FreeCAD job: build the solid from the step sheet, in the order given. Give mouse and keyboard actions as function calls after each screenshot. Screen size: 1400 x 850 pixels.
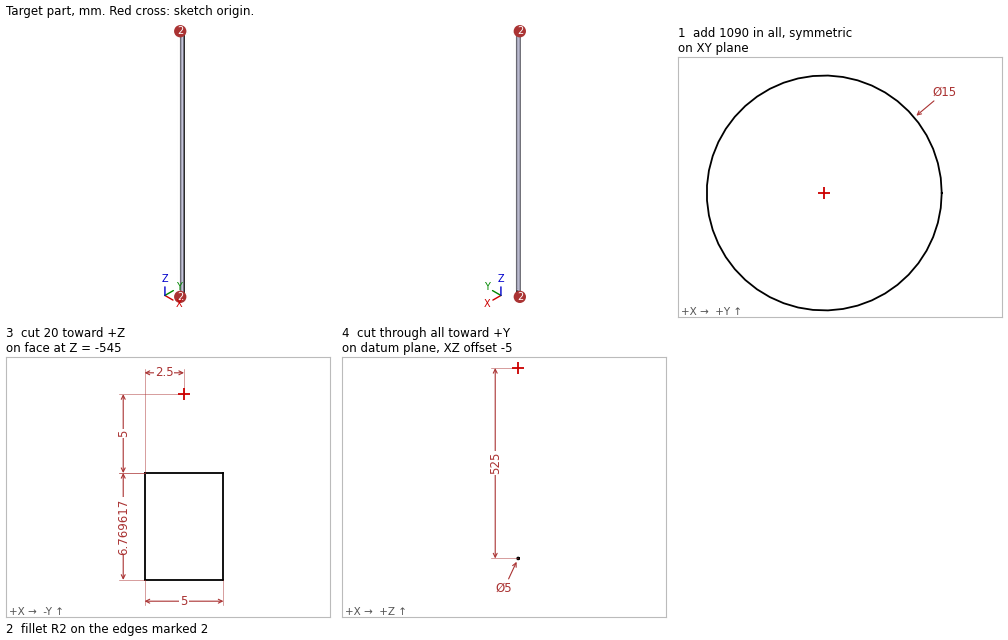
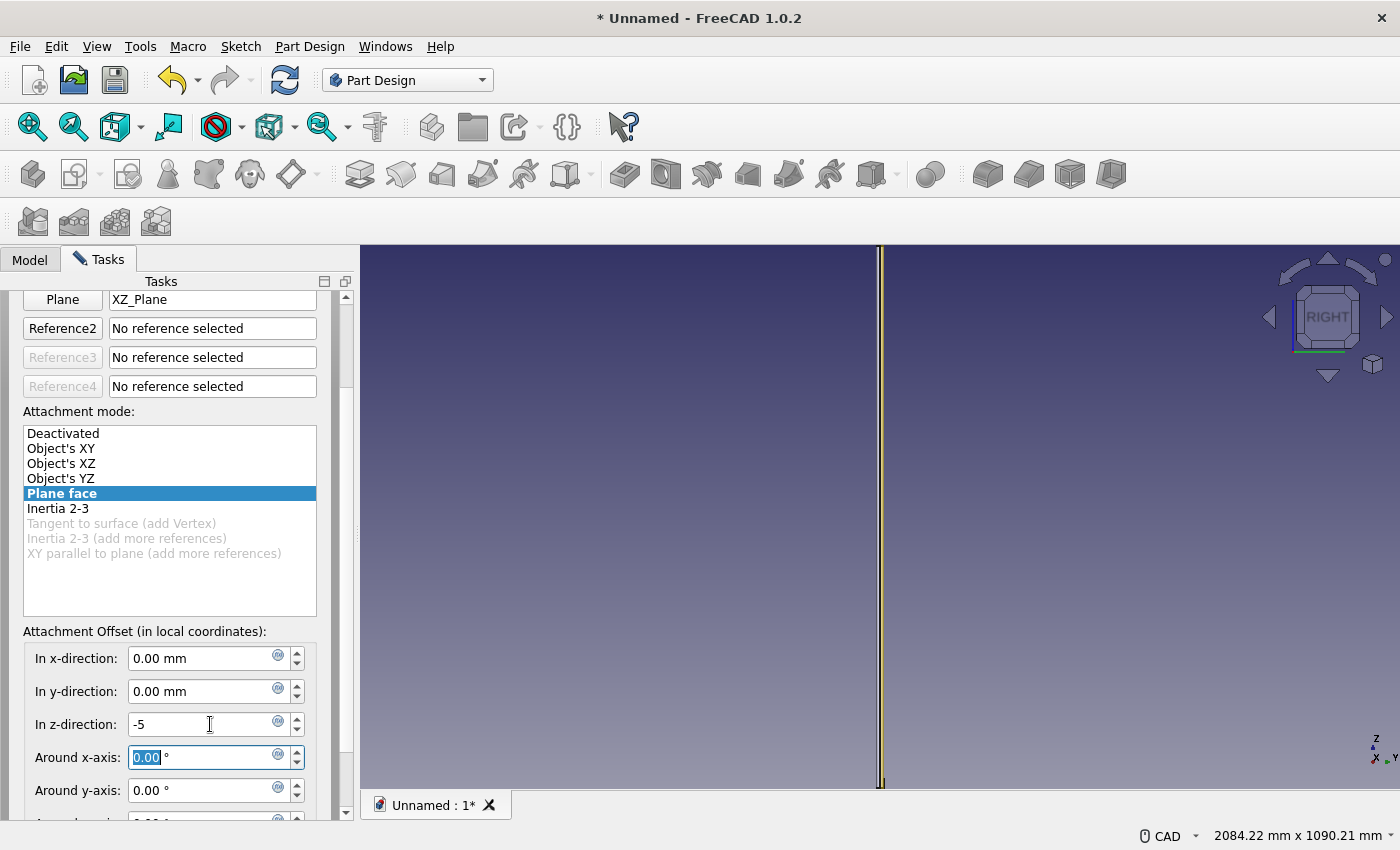
scroll(346, 556, up, 3)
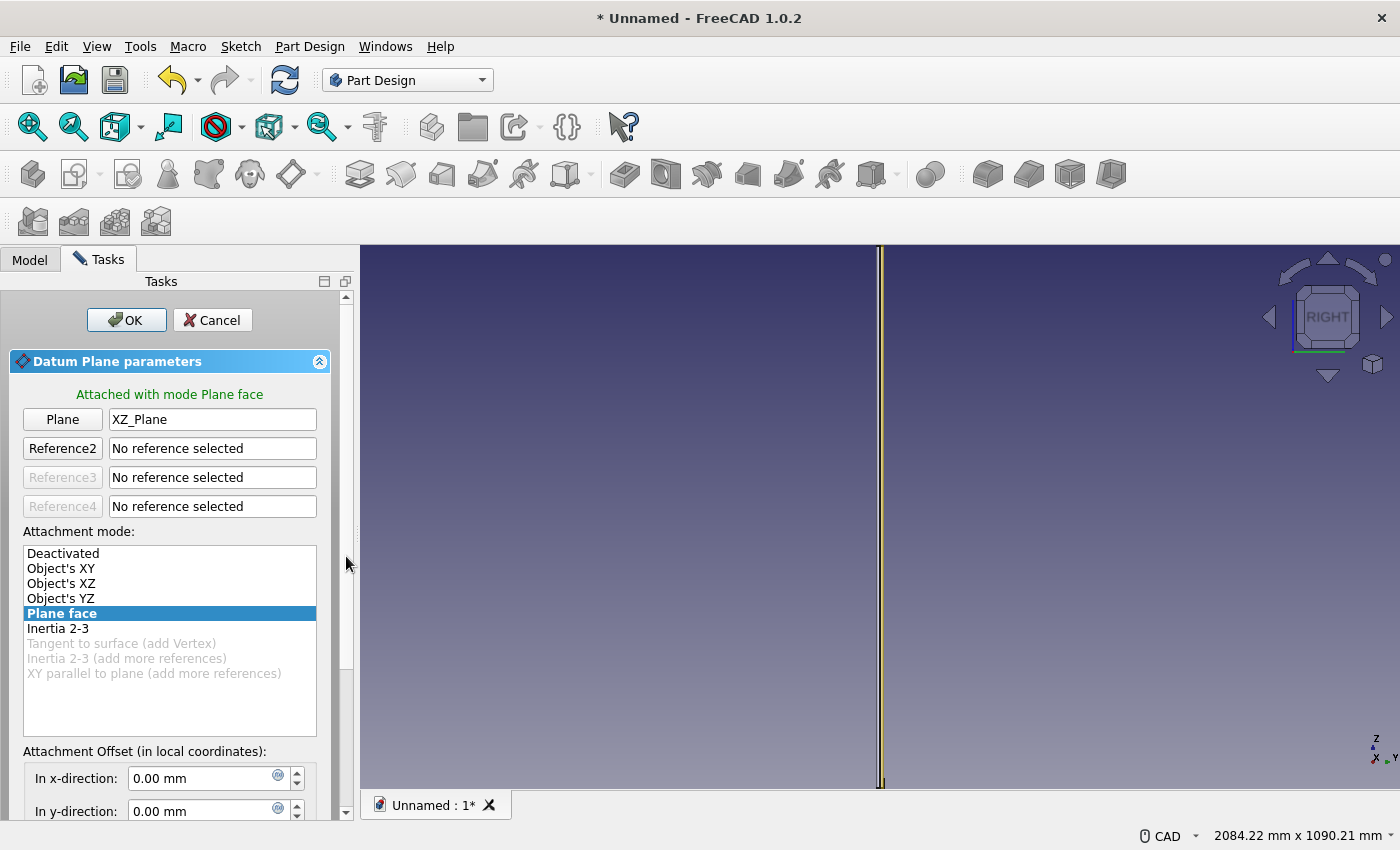
click(127, 320)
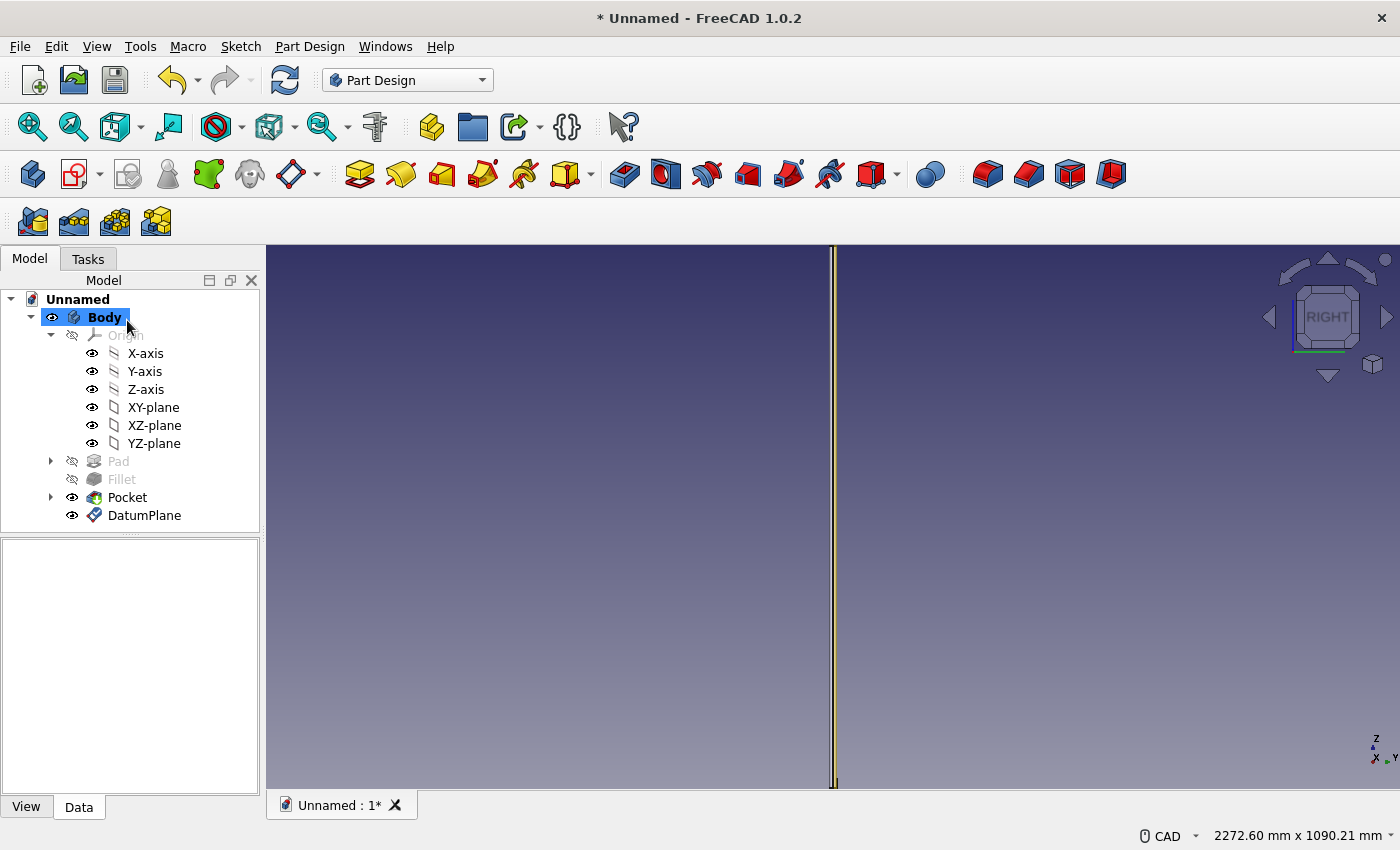
click(117, 515)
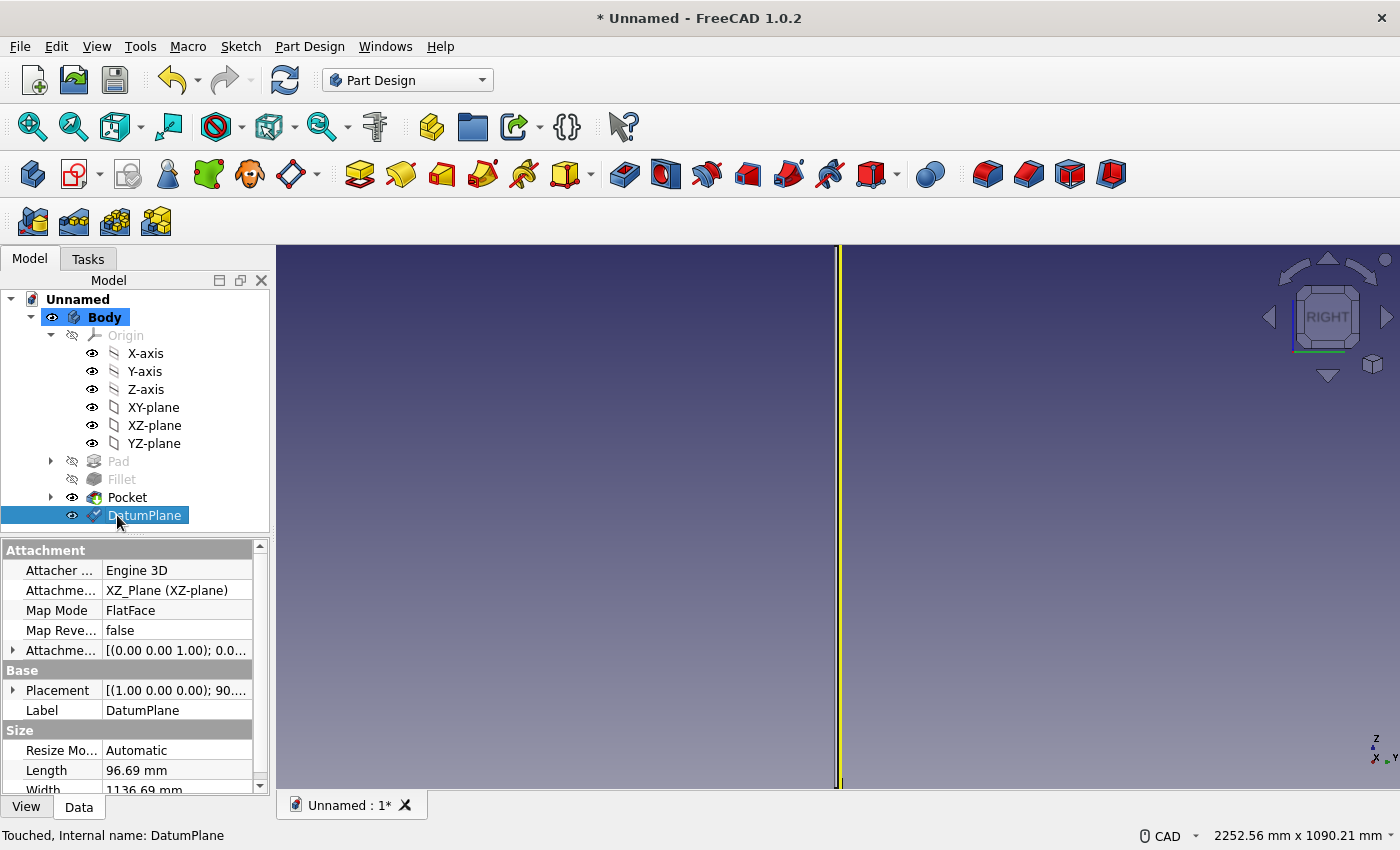
click(74, 174)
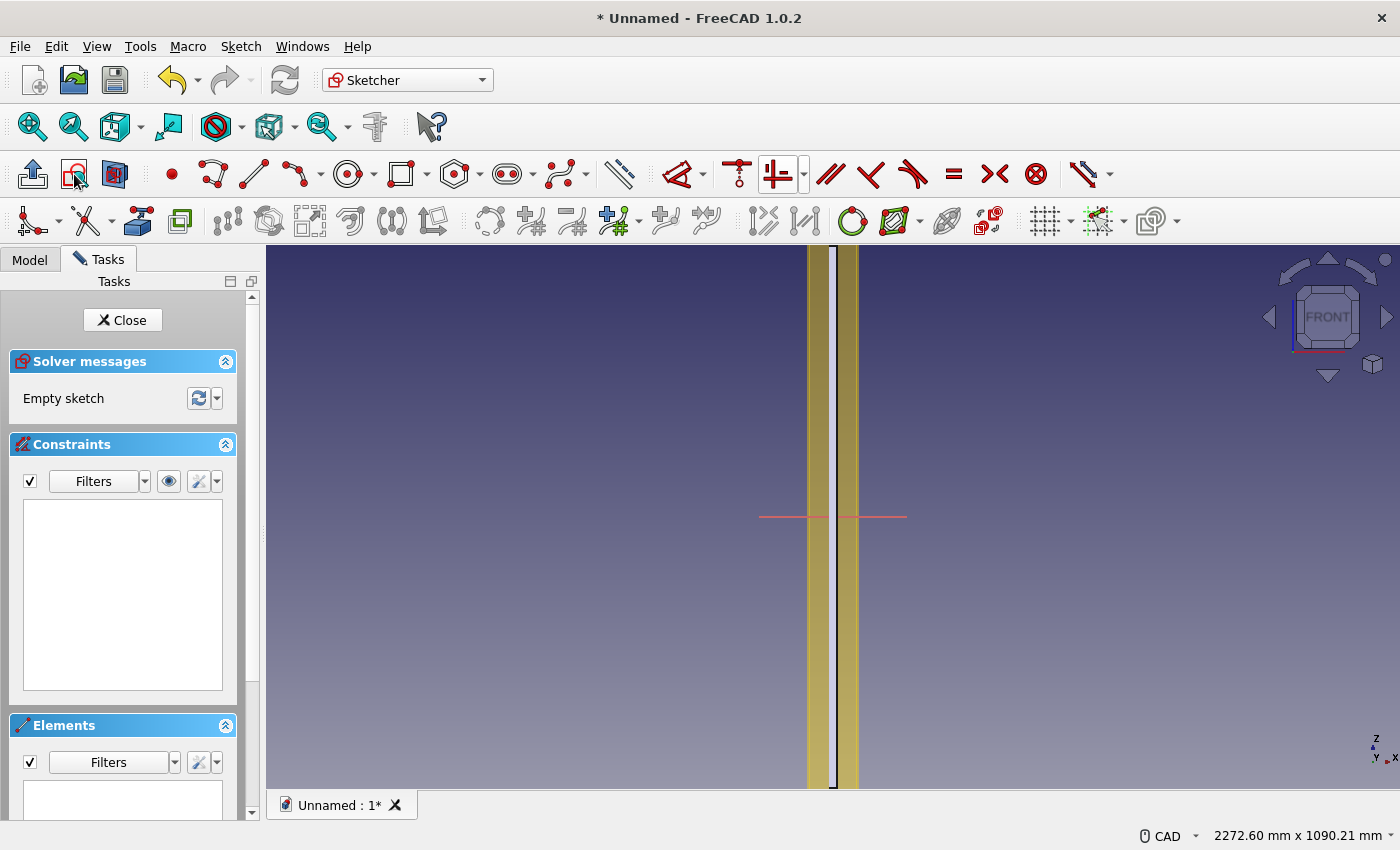
click(115, 174)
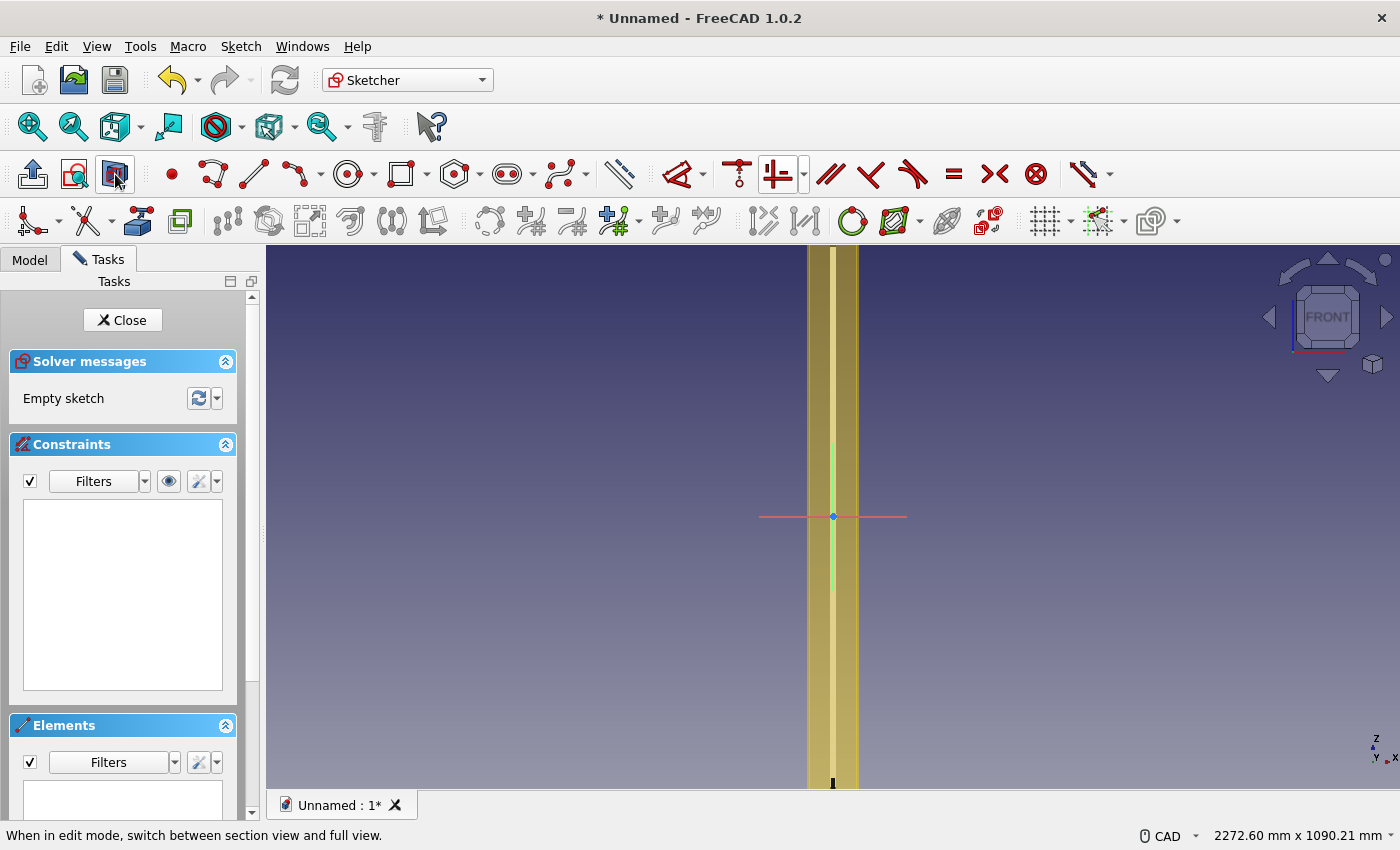
scroll(764, 517, down, 5)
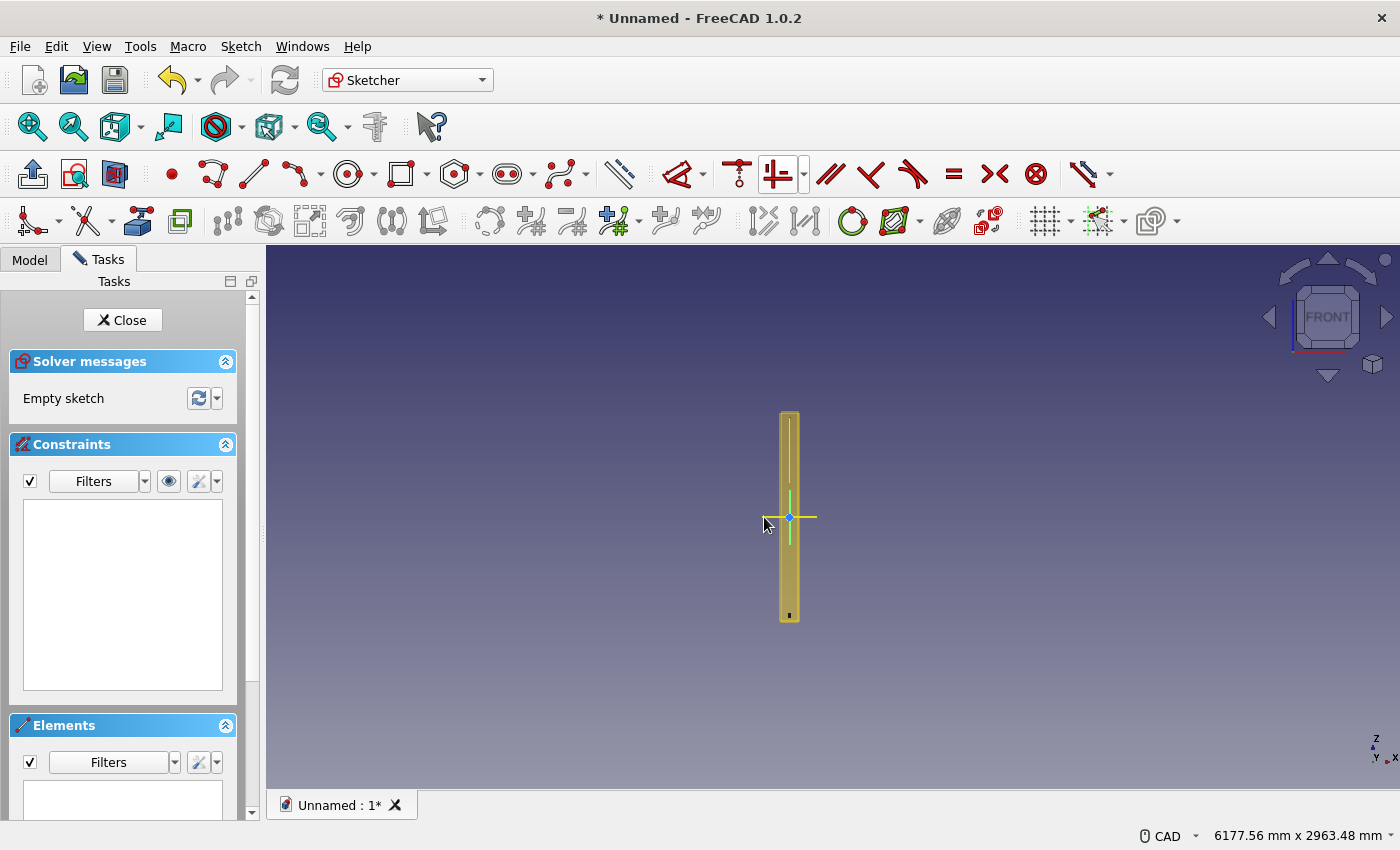
scroll(791, 619, up, 15)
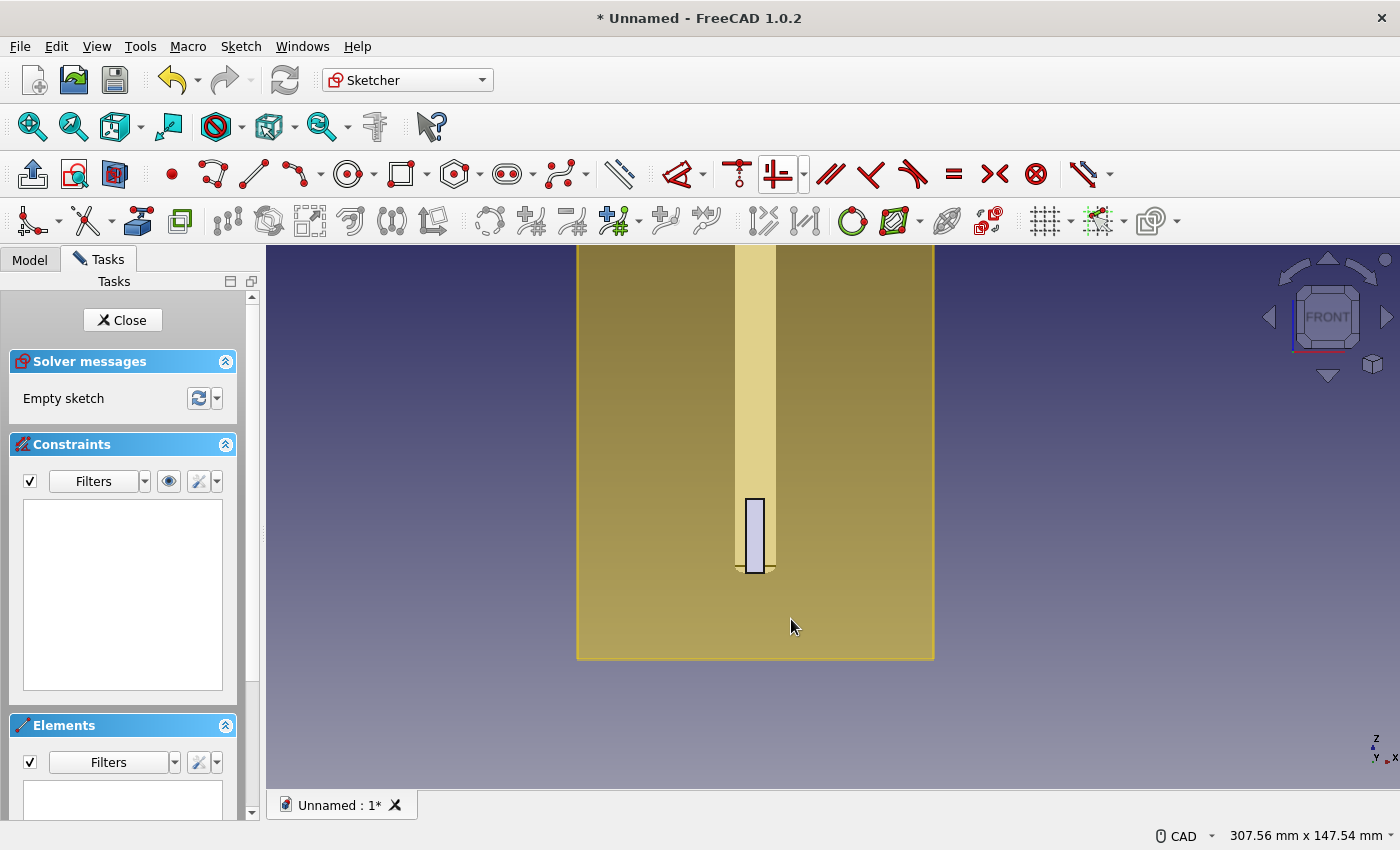
scroll(755, 498, up, 15)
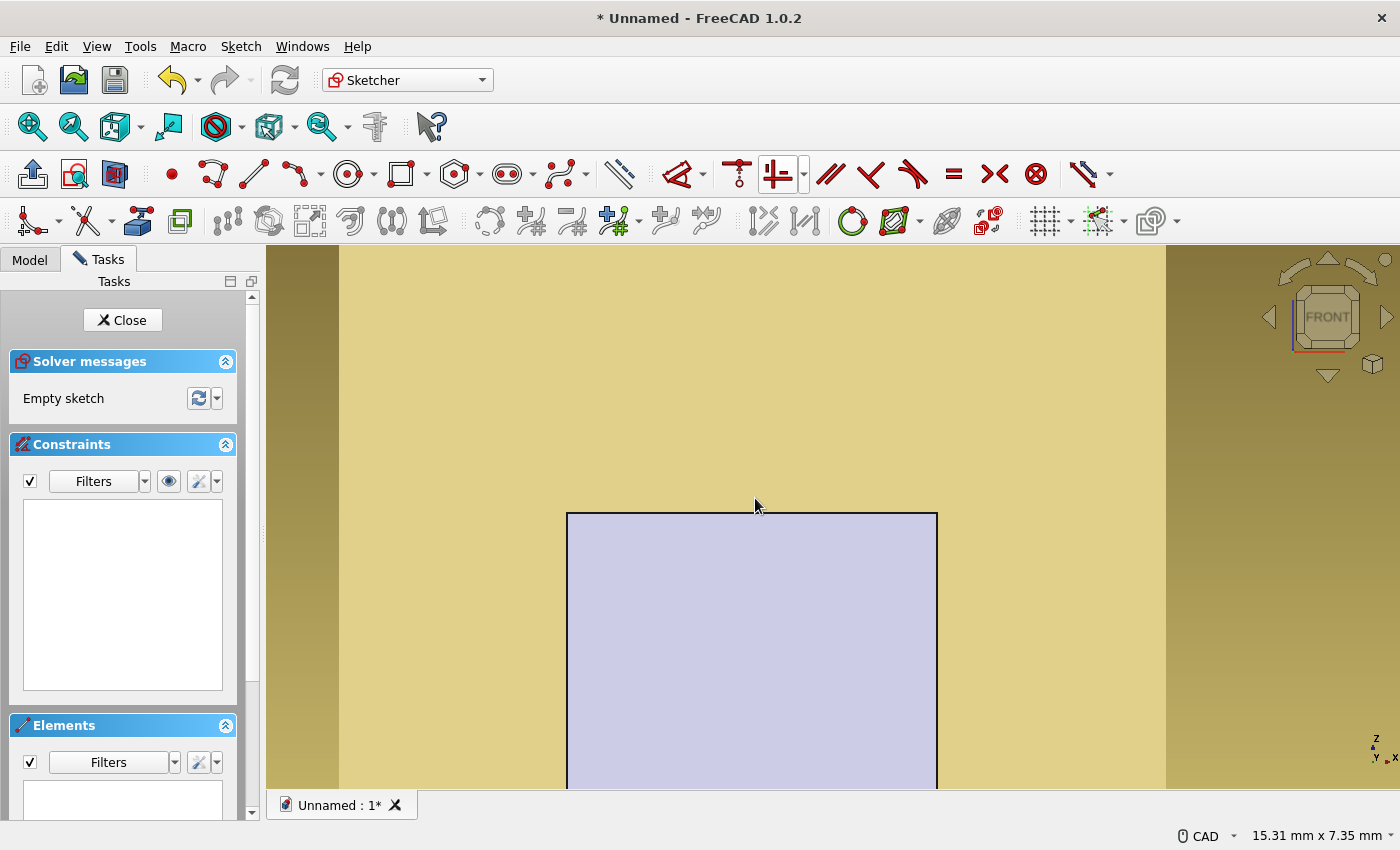
click(348, 174)